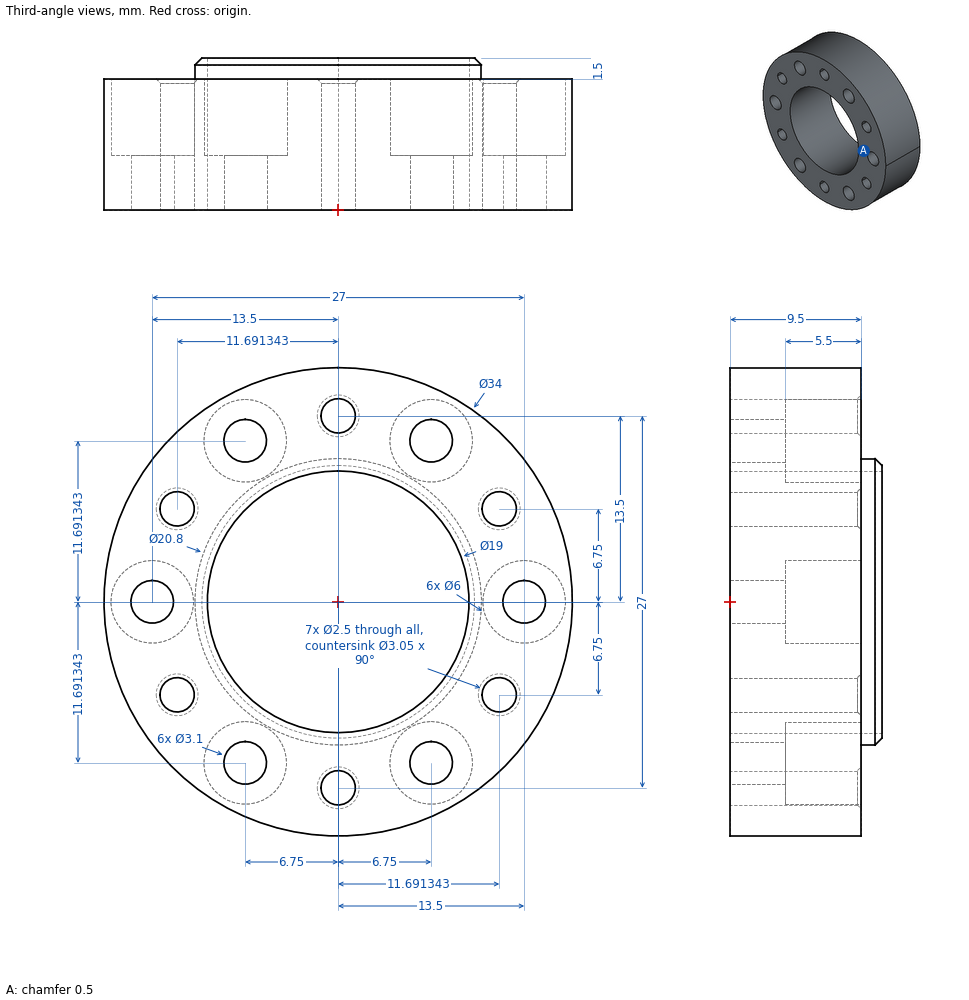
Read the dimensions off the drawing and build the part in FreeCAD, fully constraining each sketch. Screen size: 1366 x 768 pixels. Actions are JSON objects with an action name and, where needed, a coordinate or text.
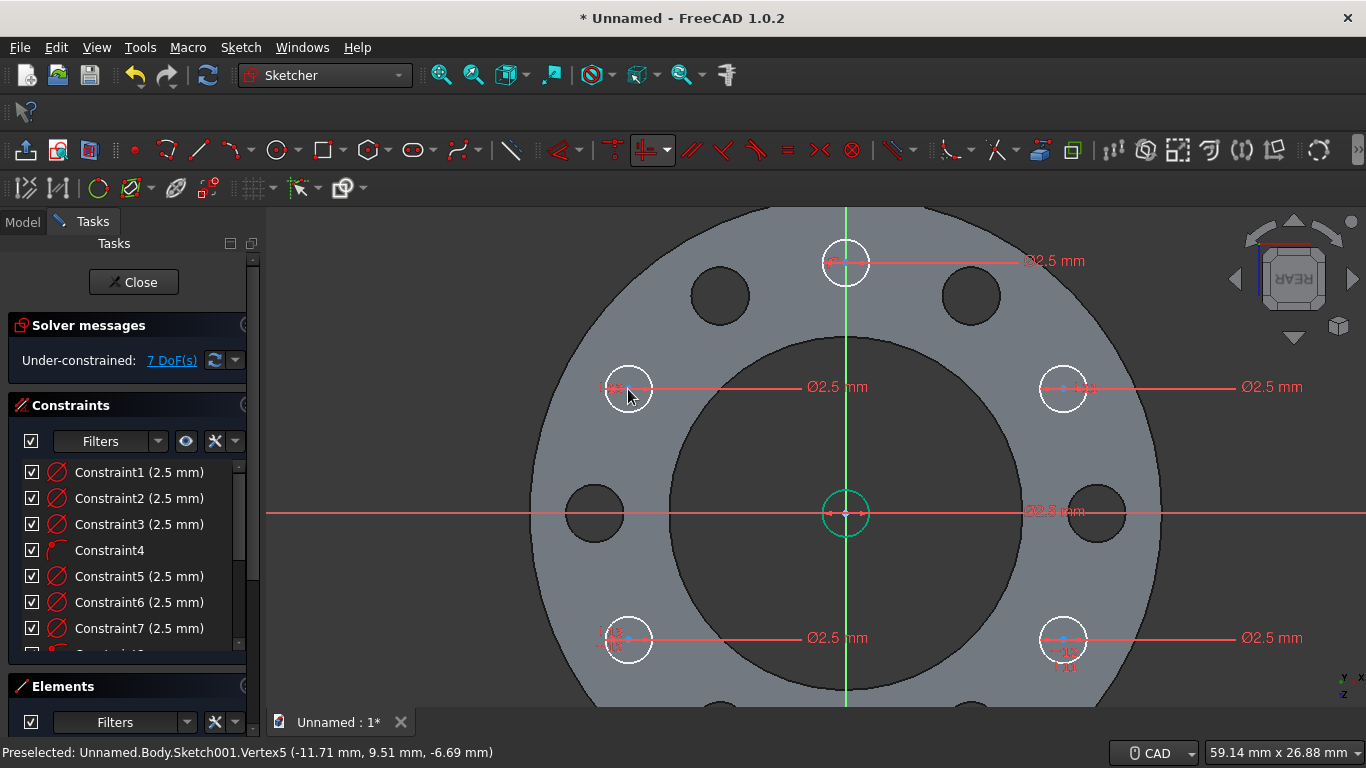
{"action": "left_click", "coordinate": [1063, 389]}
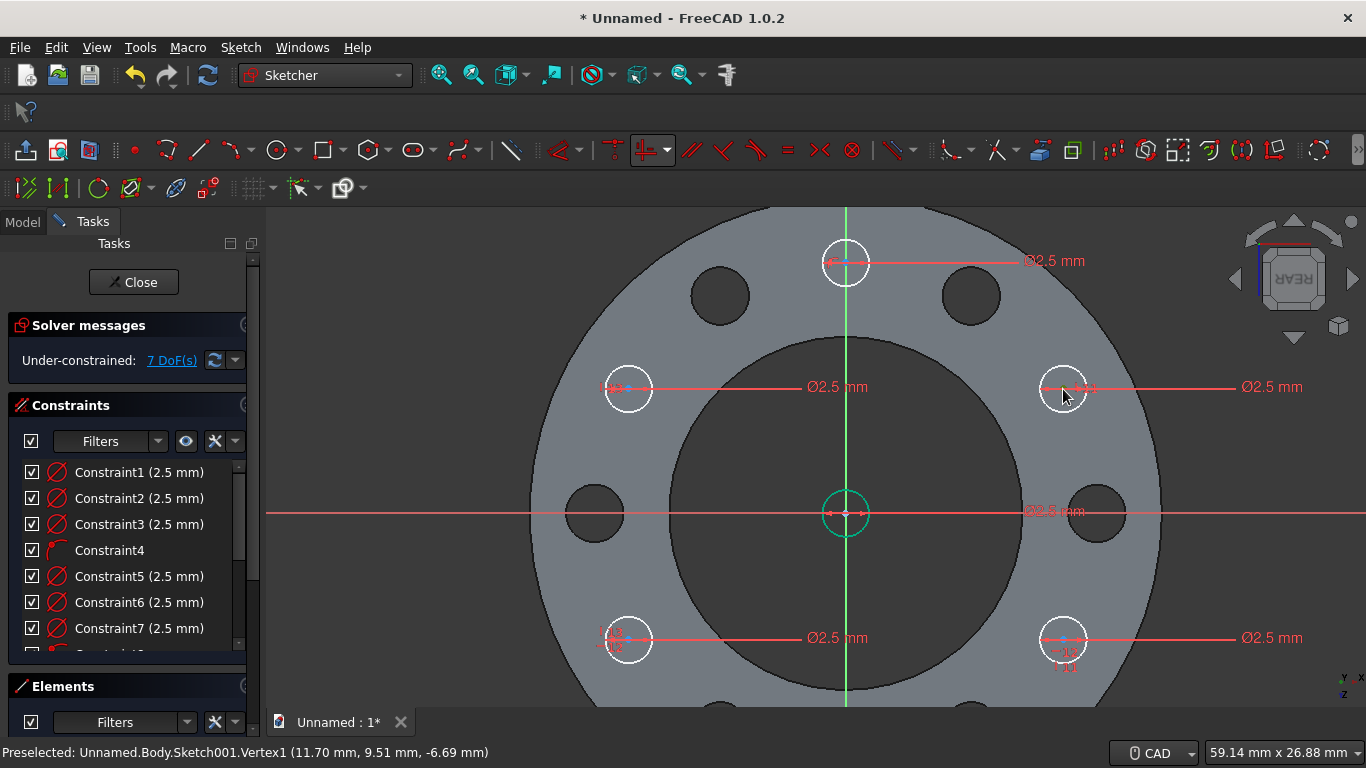
{"action": "left_click", "coordinate": [629, 389]}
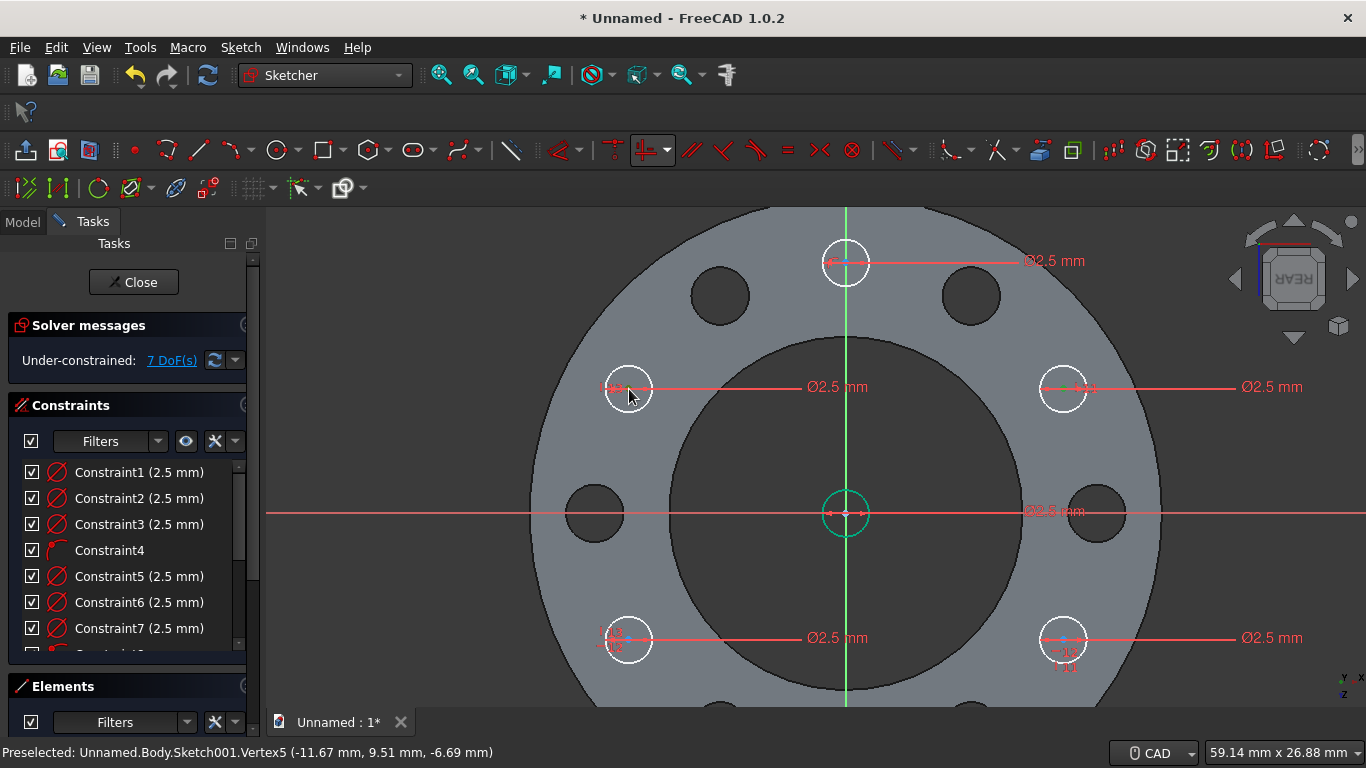
{"action": "key", "text": "h"}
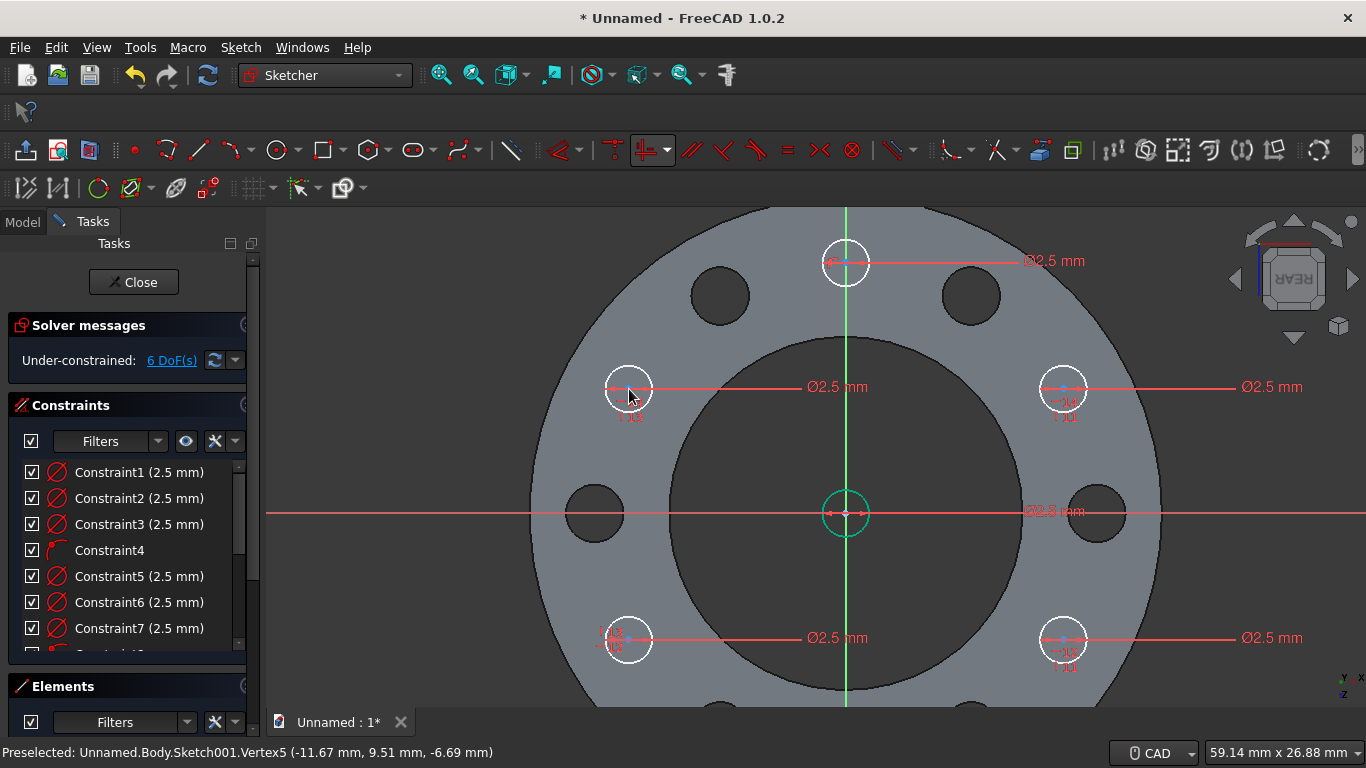
{"action": "left_click", "coordinate": [558, 150]}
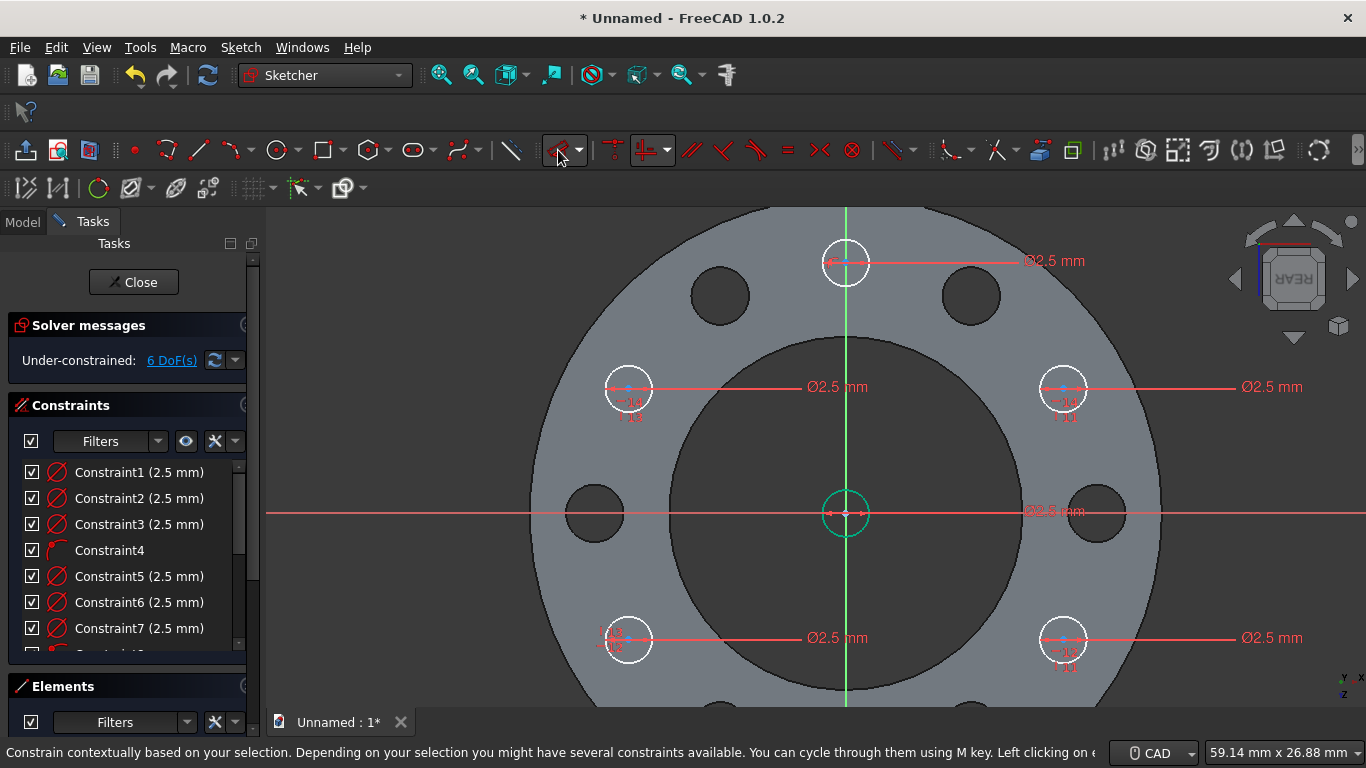
{"action": "scroll", "coordinate": [628, 388], "scroll_direction": "down", "scroll_amount": 3}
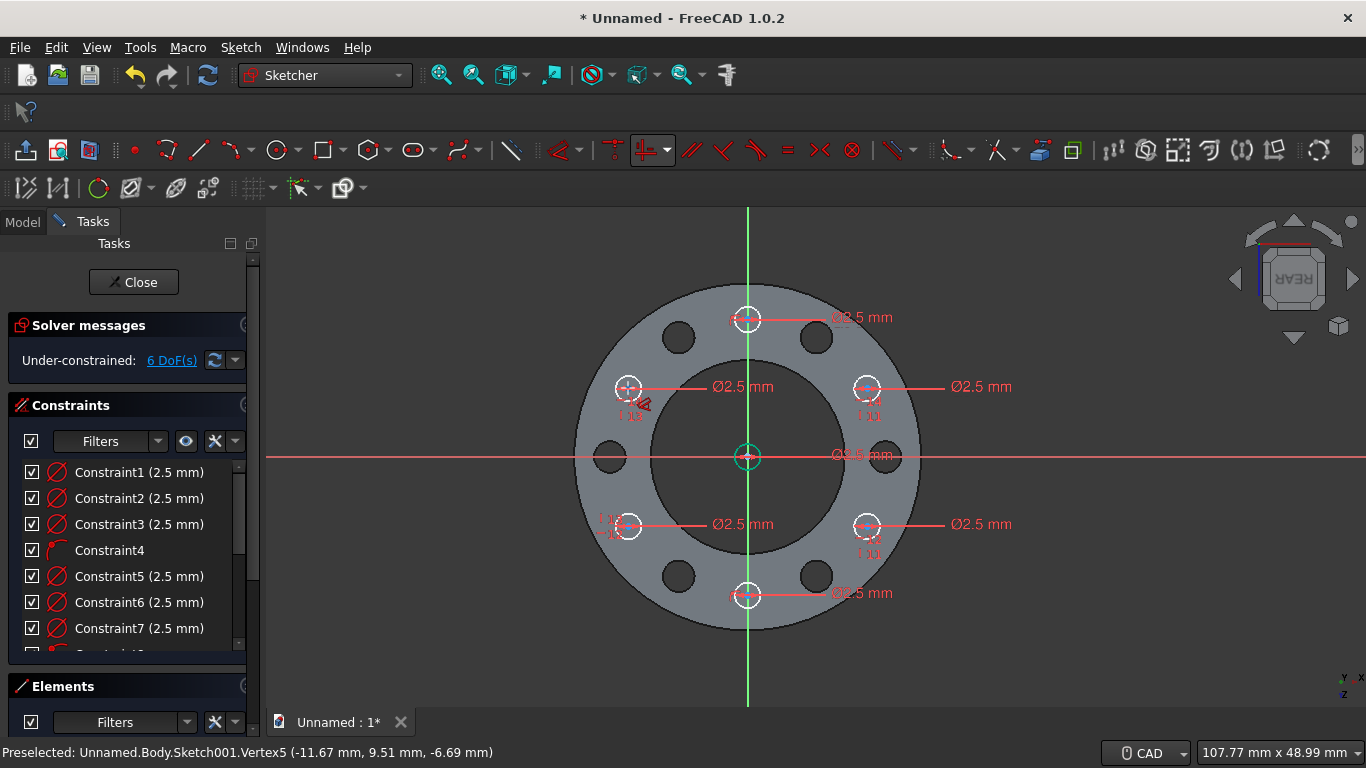
{"action": "left_click", "coordinate": [748, 595]}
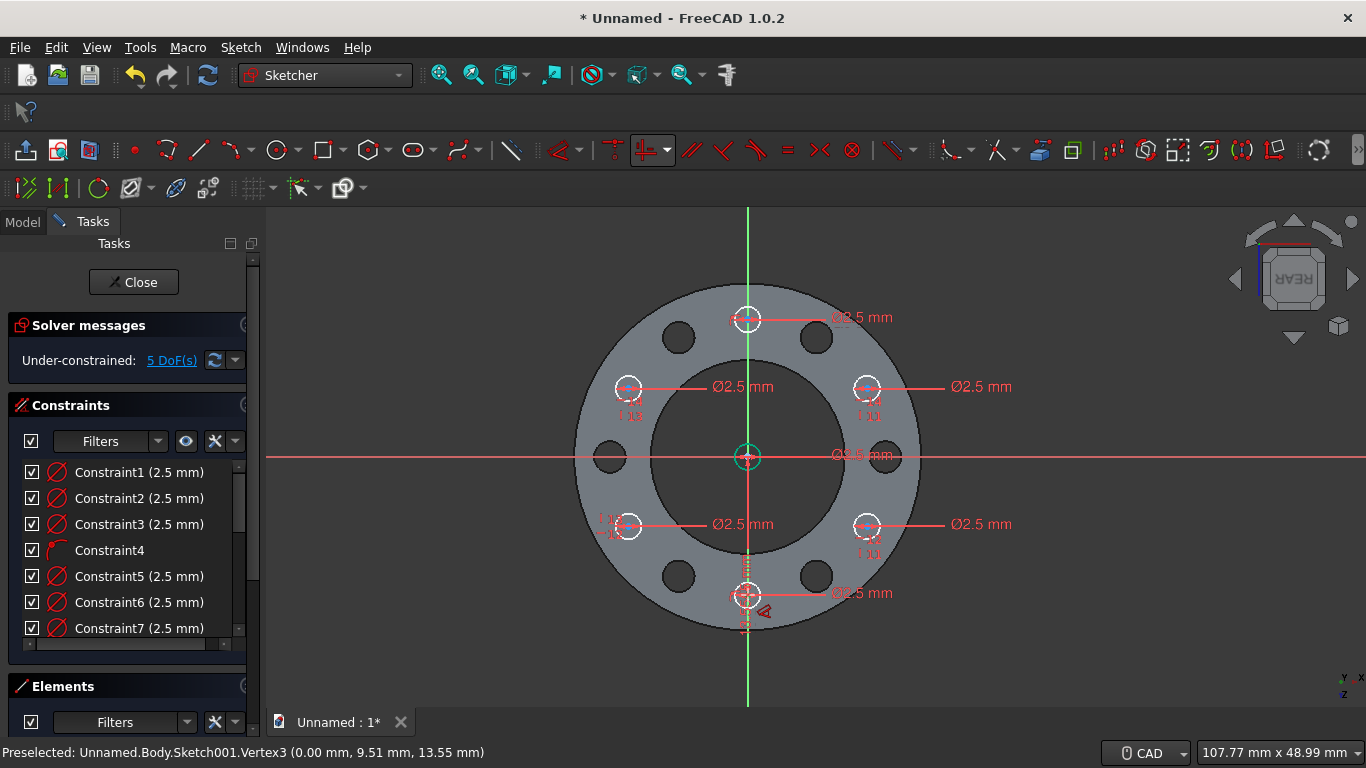
{"action": "left_click", "coordinate": [748, 320]}
{"action": "left_click", "coordinate": [782, 394]}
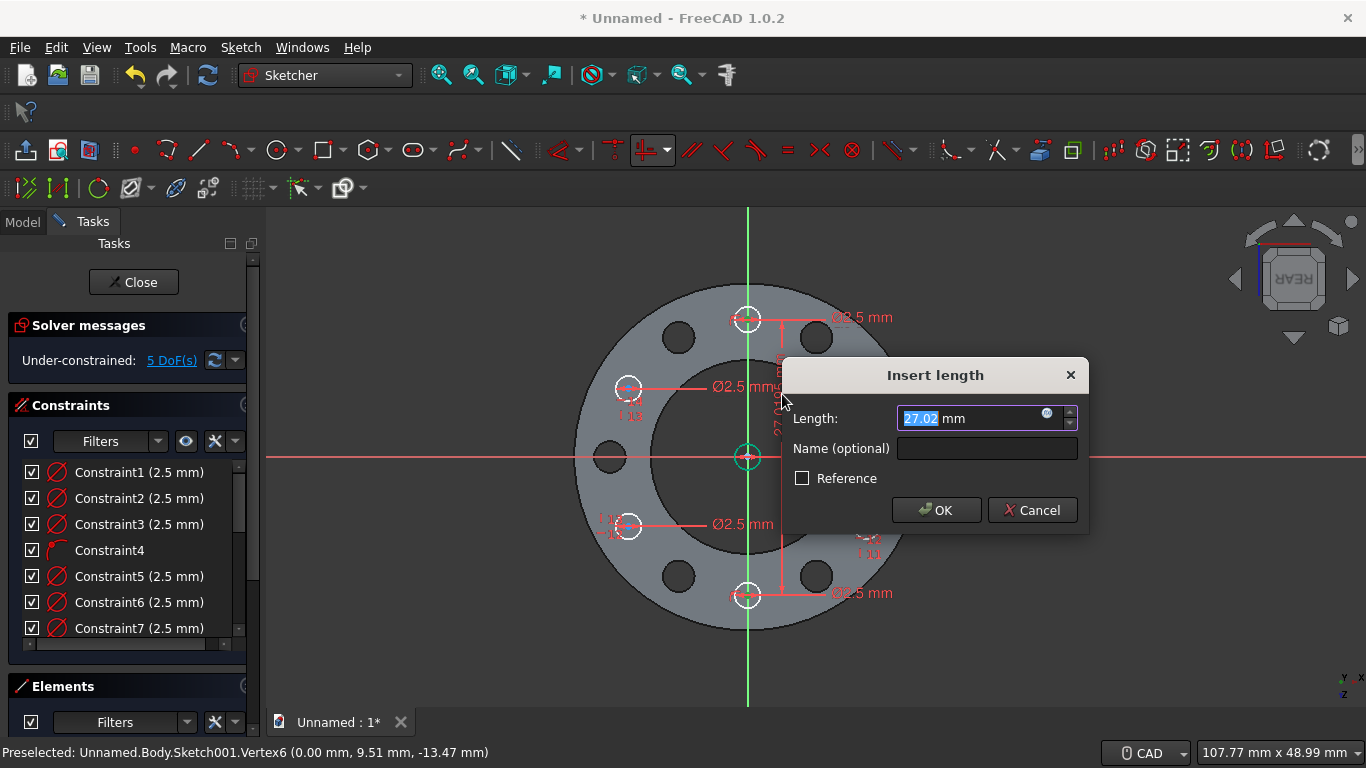
{"action": "type", "text": "27"}
{"action": "key", "text": "Return"}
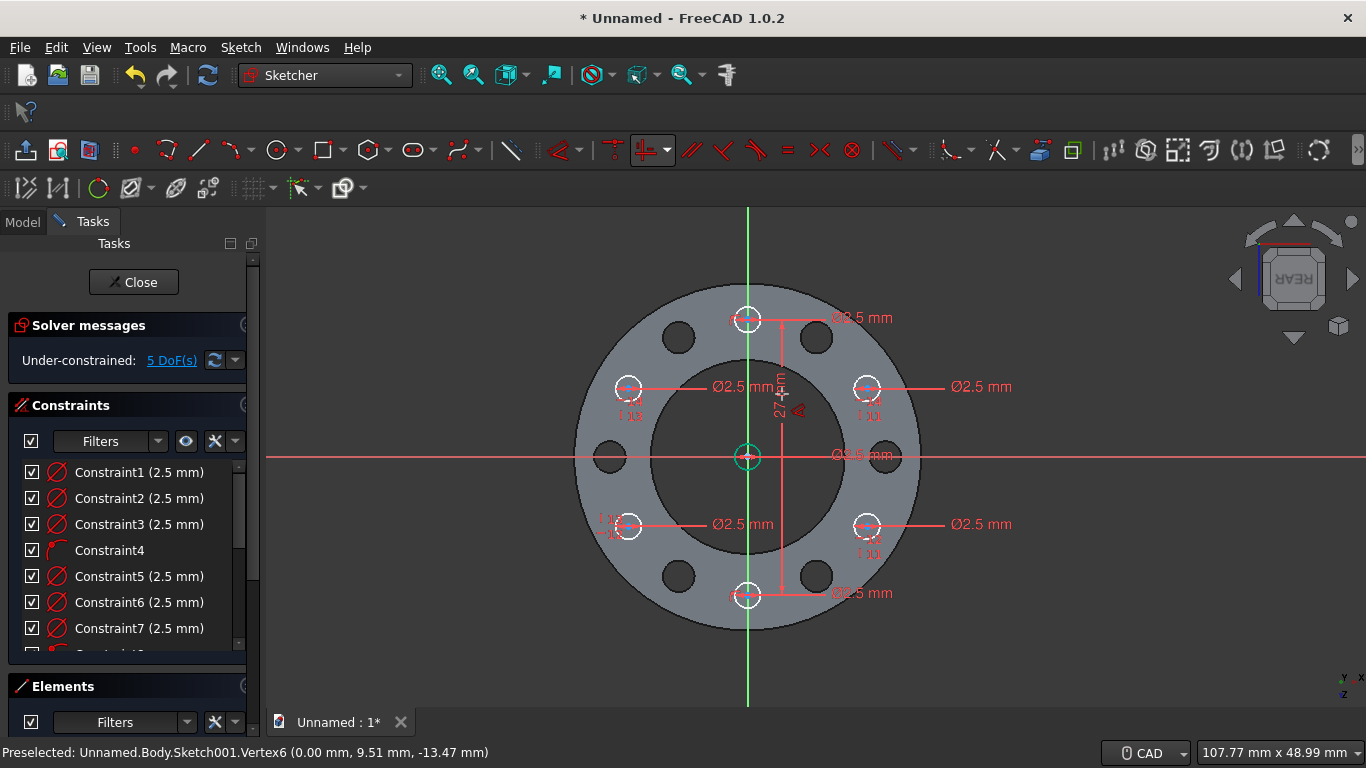
{"action": "left_click", "coordinate": [867, 389]}
{"action": "left_click", "coordinate": [901, 423]}